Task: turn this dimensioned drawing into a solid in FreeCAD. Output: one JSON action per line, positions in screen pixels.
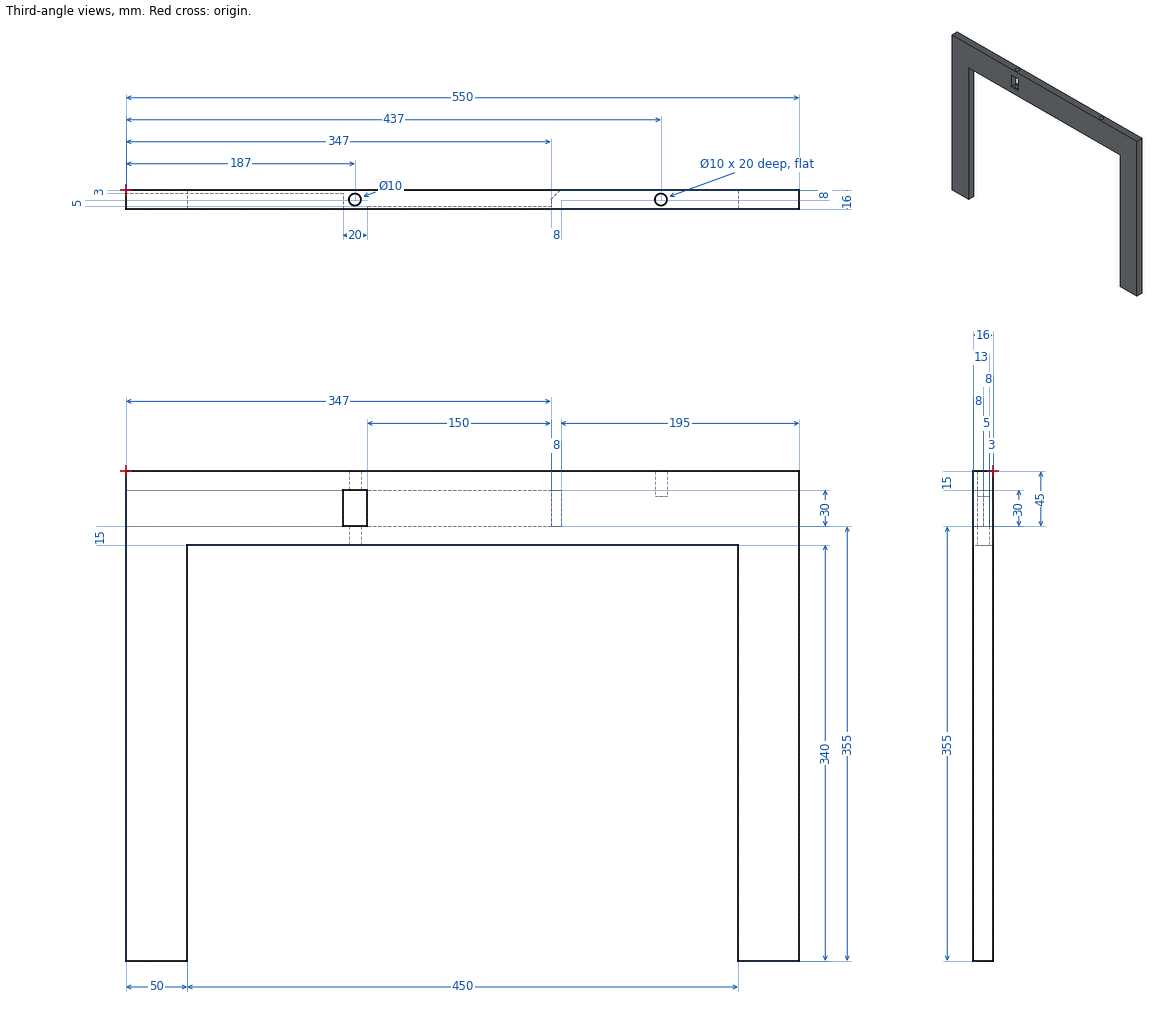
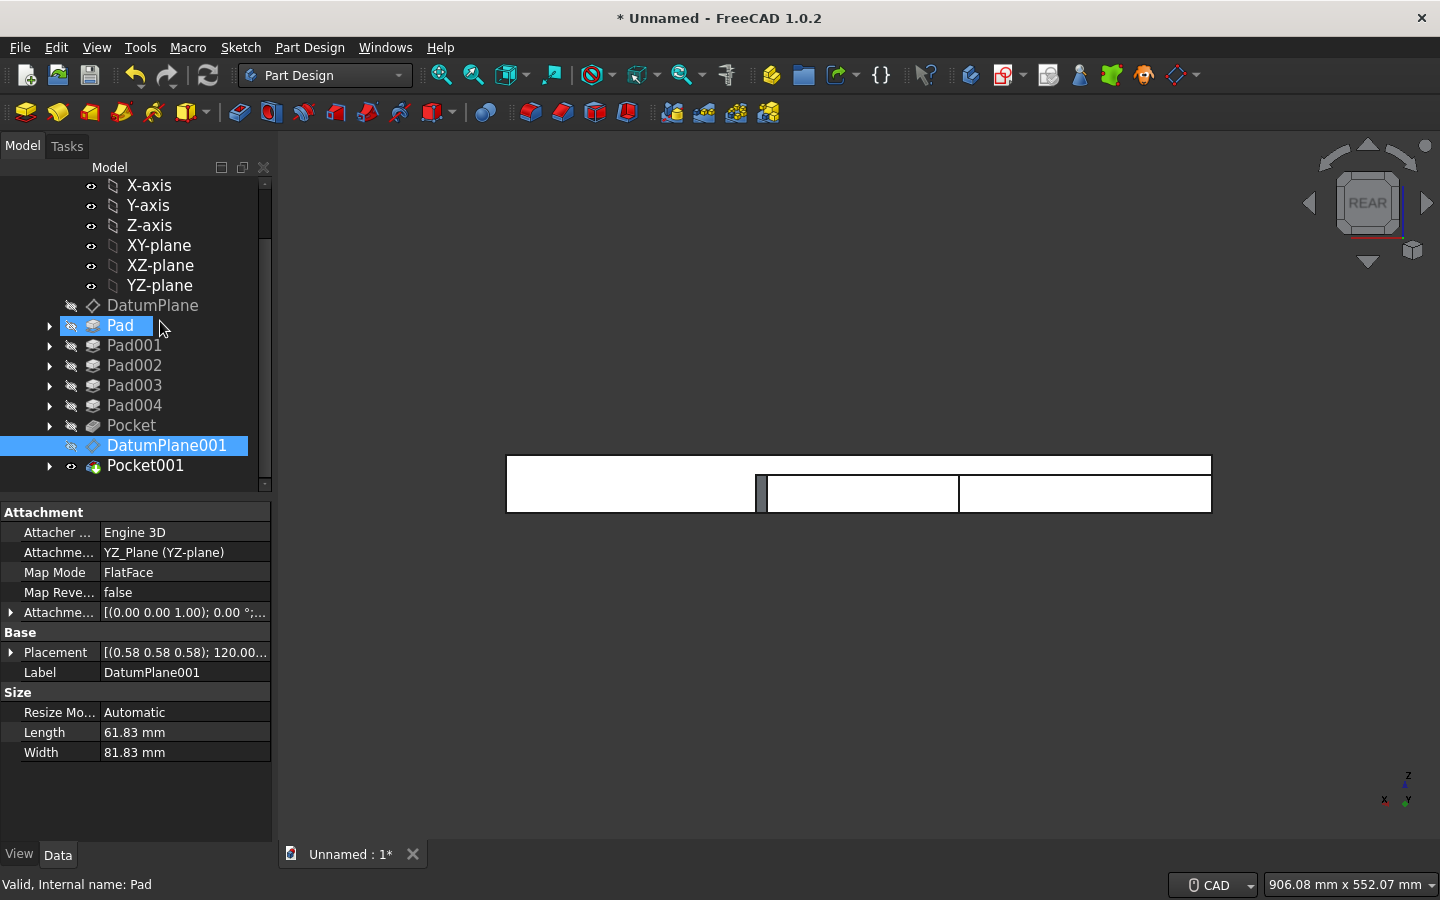
{"action": "scroll", "coordinate": [160, 321], "scroll_direction": "up", "scroll_amount": 15}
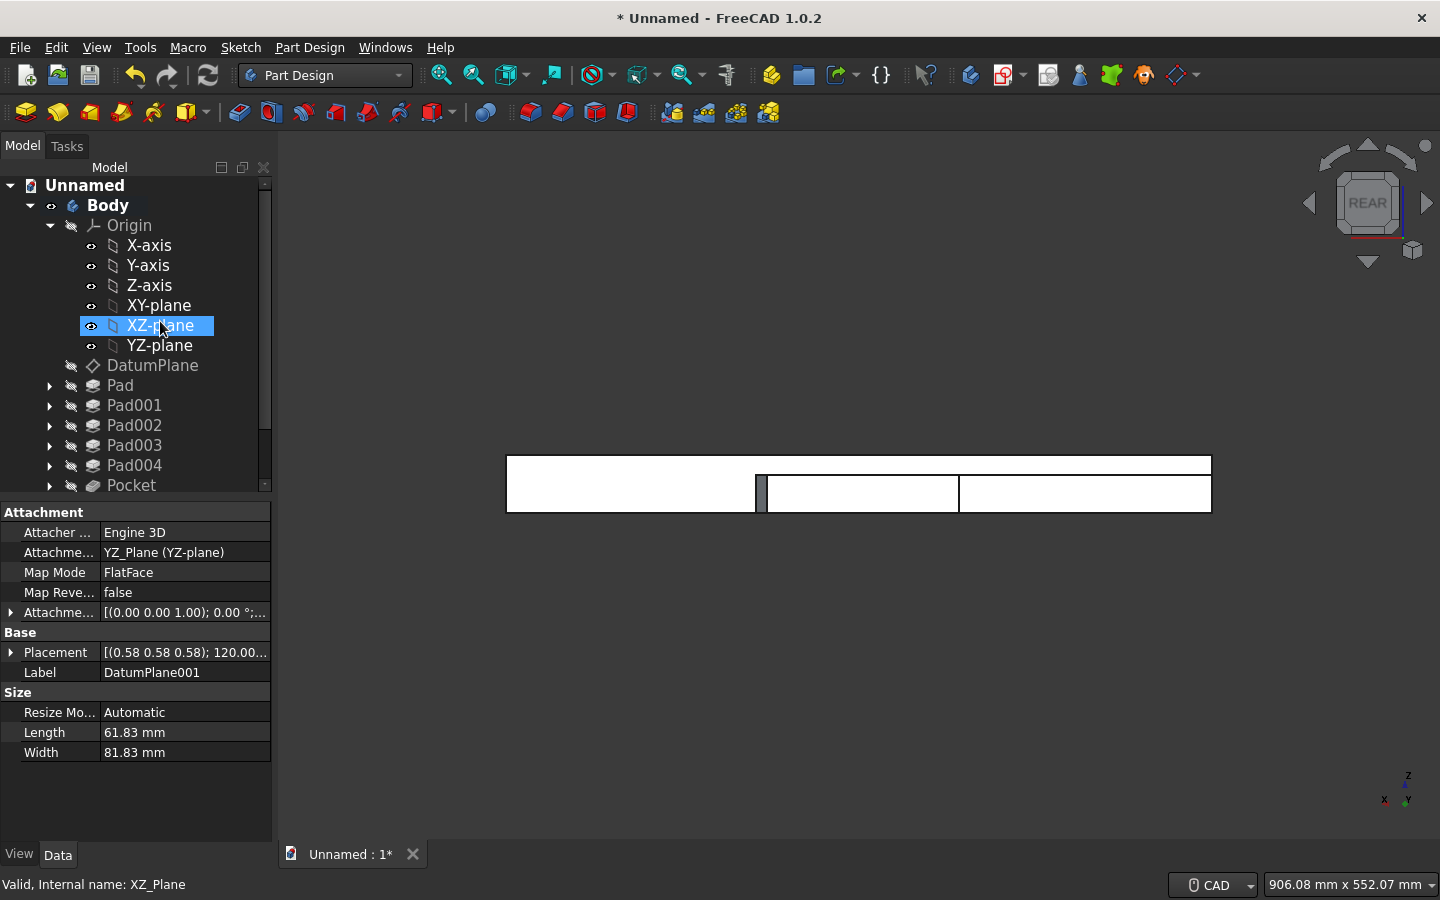
{"action": "left_click", "coordinate": [136, 346]}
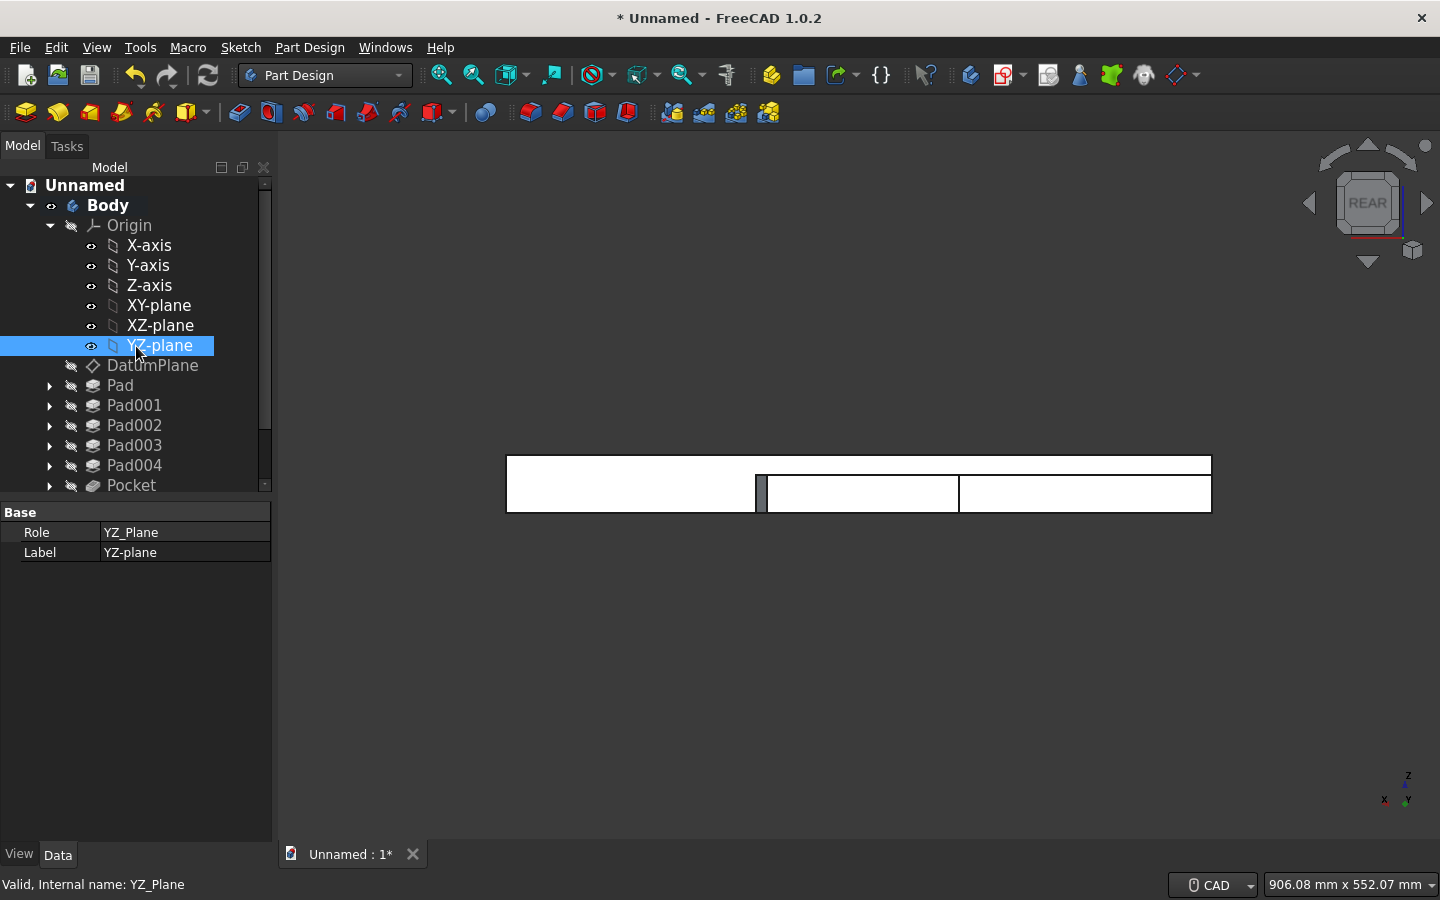
{"action": "left_click", "coordinate": [1176, 76]}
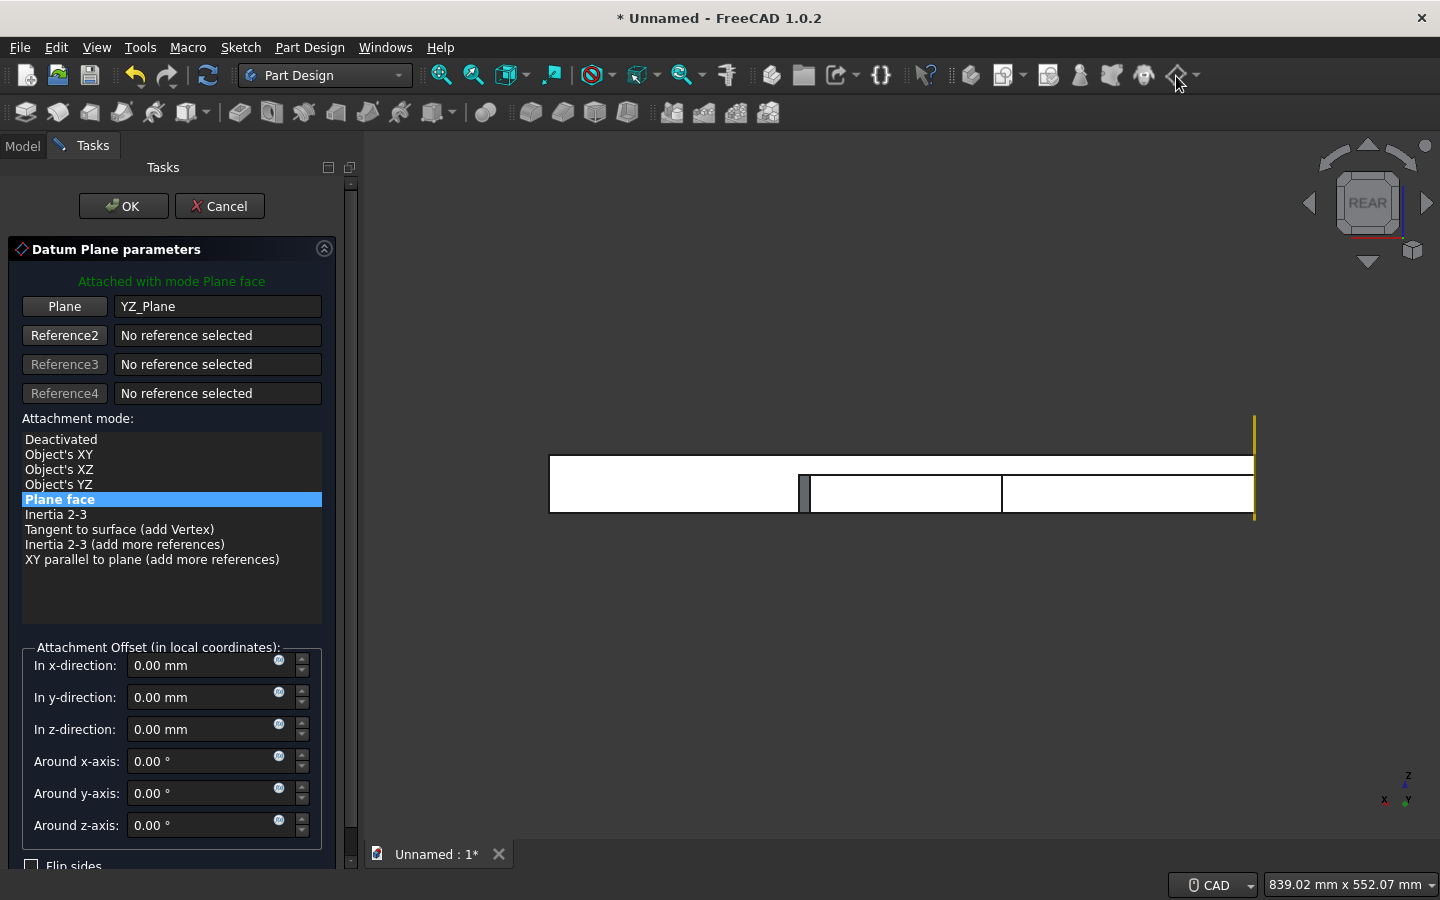
{"action": "triple_click", "coordinate": [210, 729]}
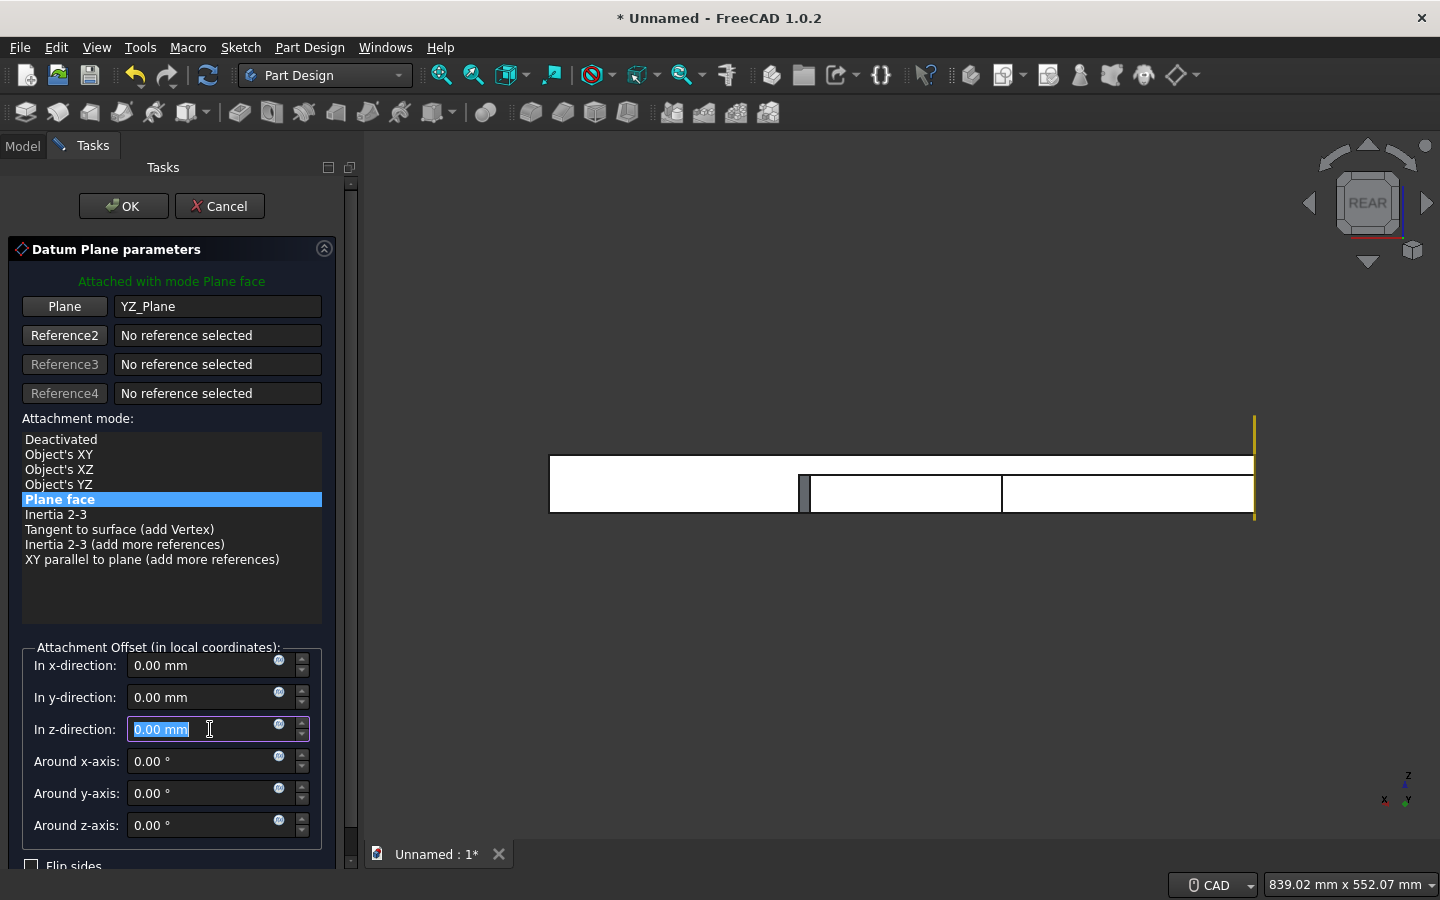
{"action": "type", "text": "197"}
{"action": "key", "text": "Tab"}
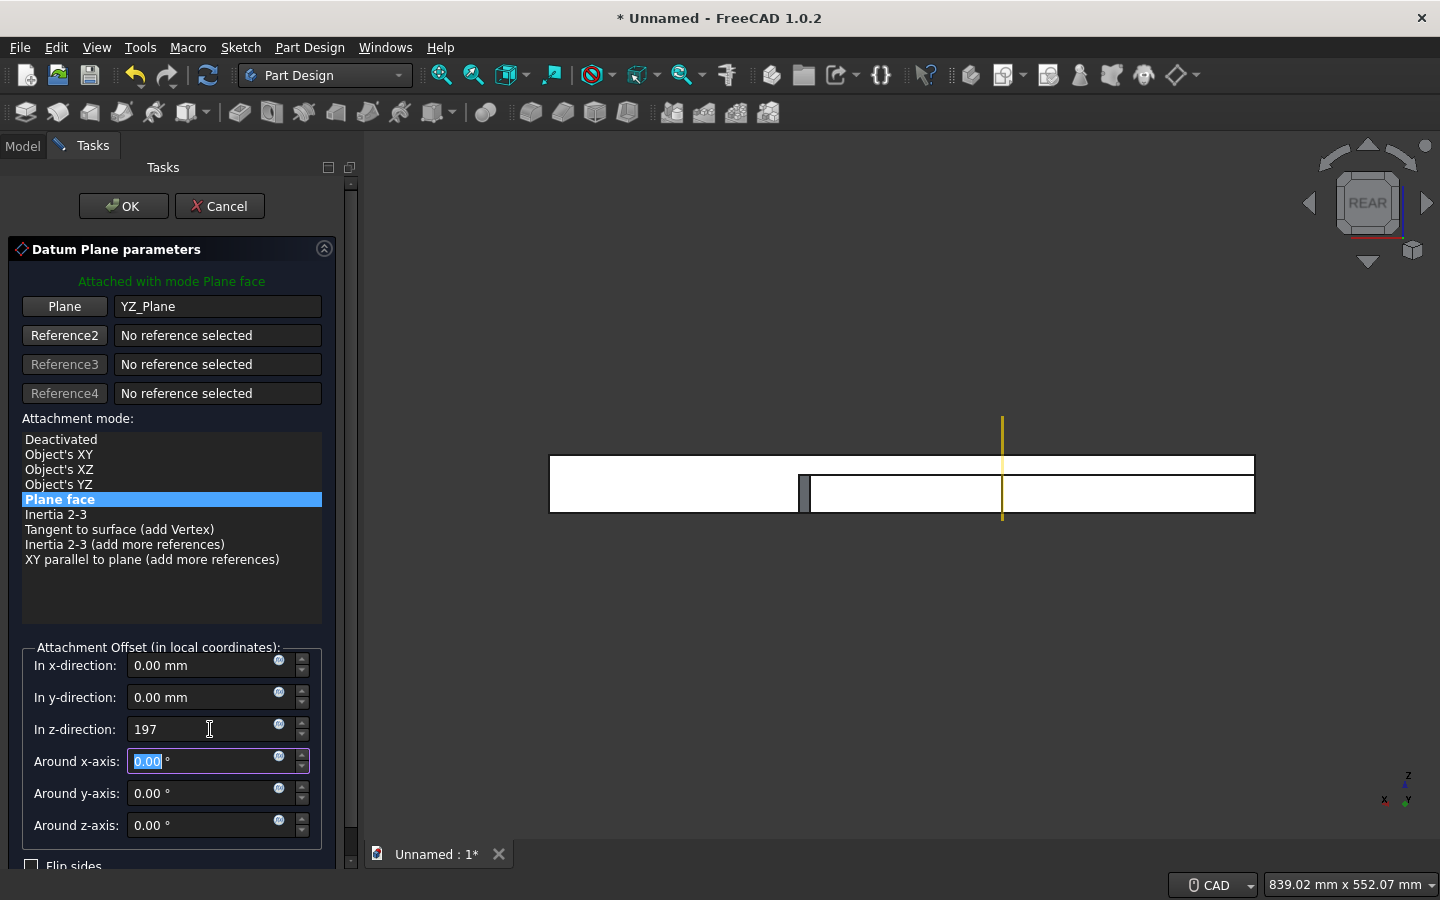
{"action": "left_click", "coordinate": [124, 206]}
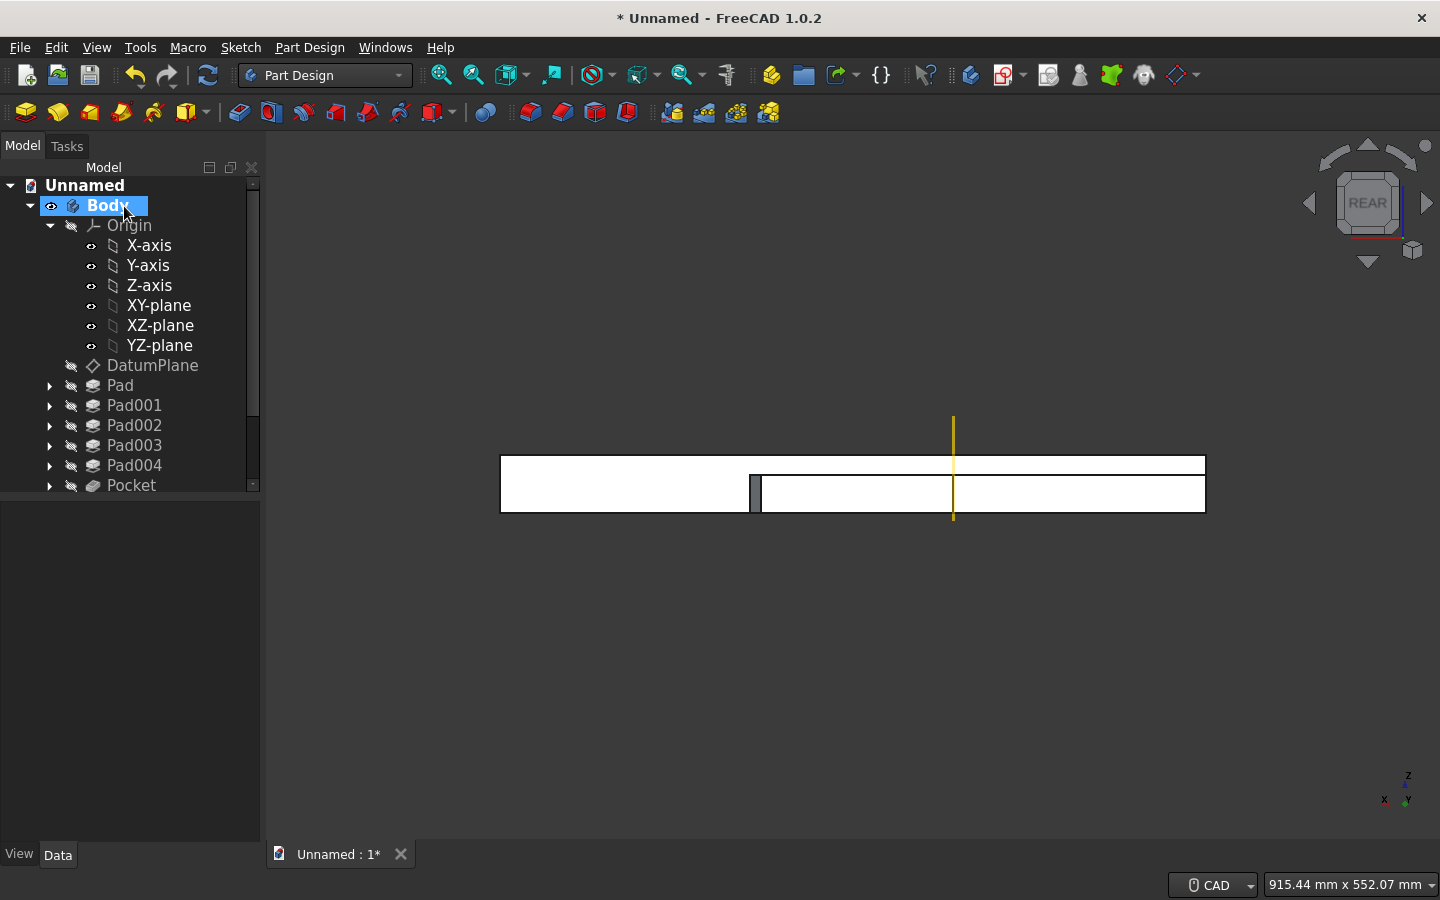
{"action": "scroll", "coordinate": [100, 341], "scroll_direction": "down", "scroll_amount": 3}